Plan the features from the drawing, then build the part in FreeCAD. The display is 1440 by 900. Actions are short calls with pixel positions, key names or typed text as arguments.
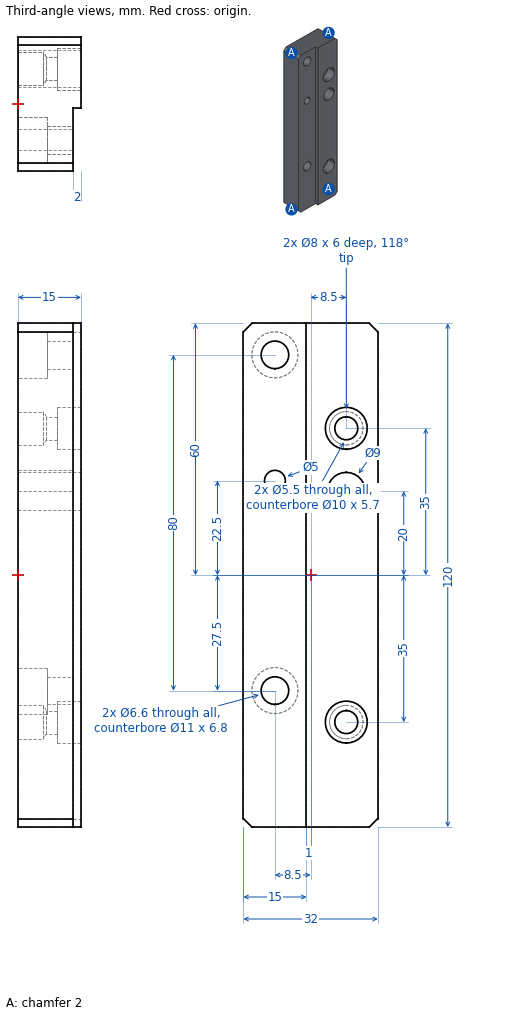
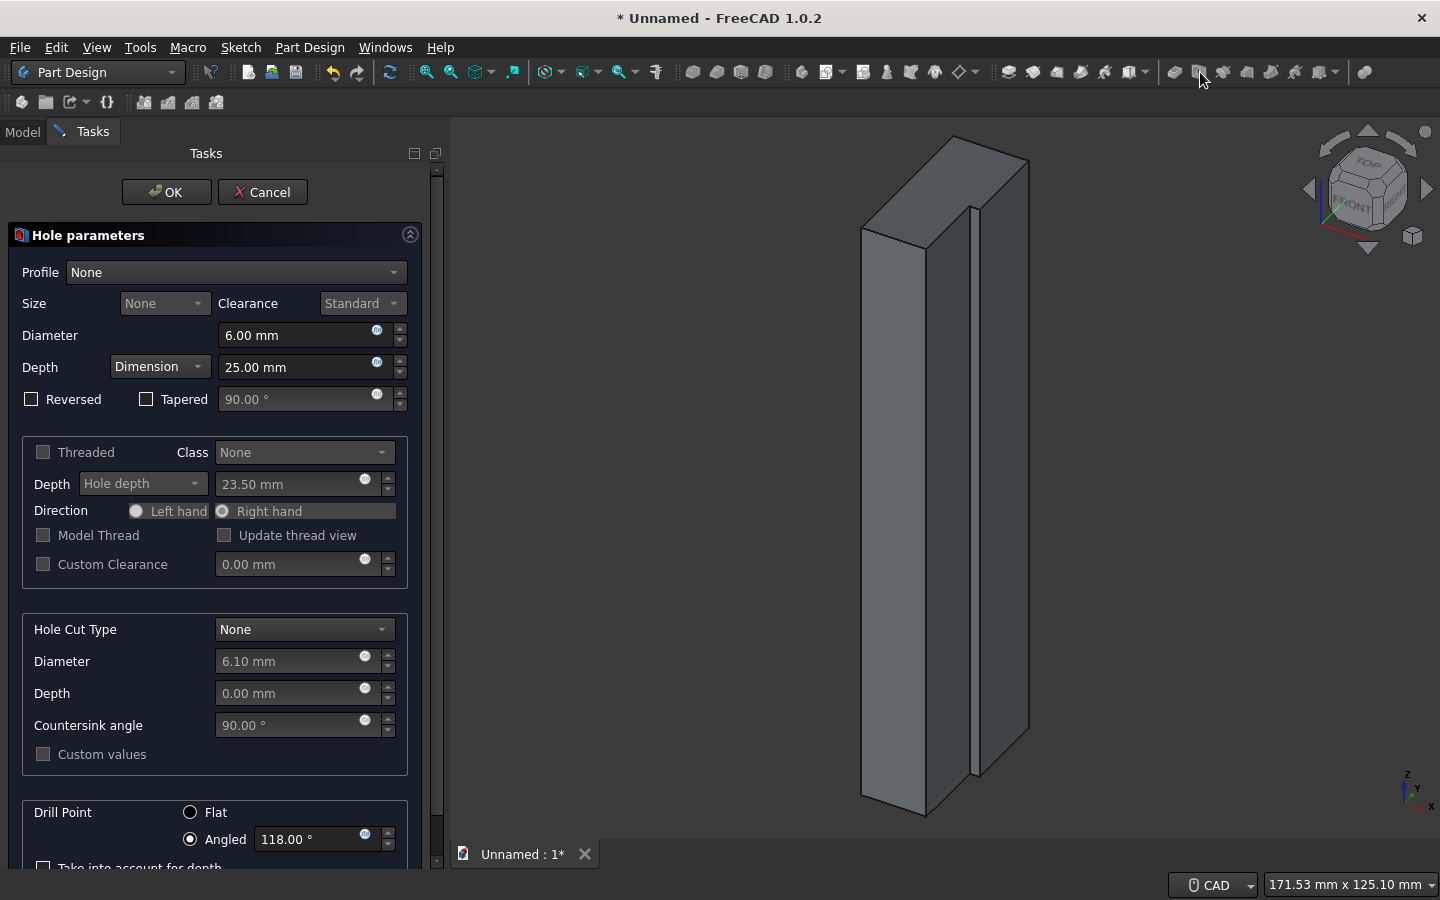
triple_click(305, 335)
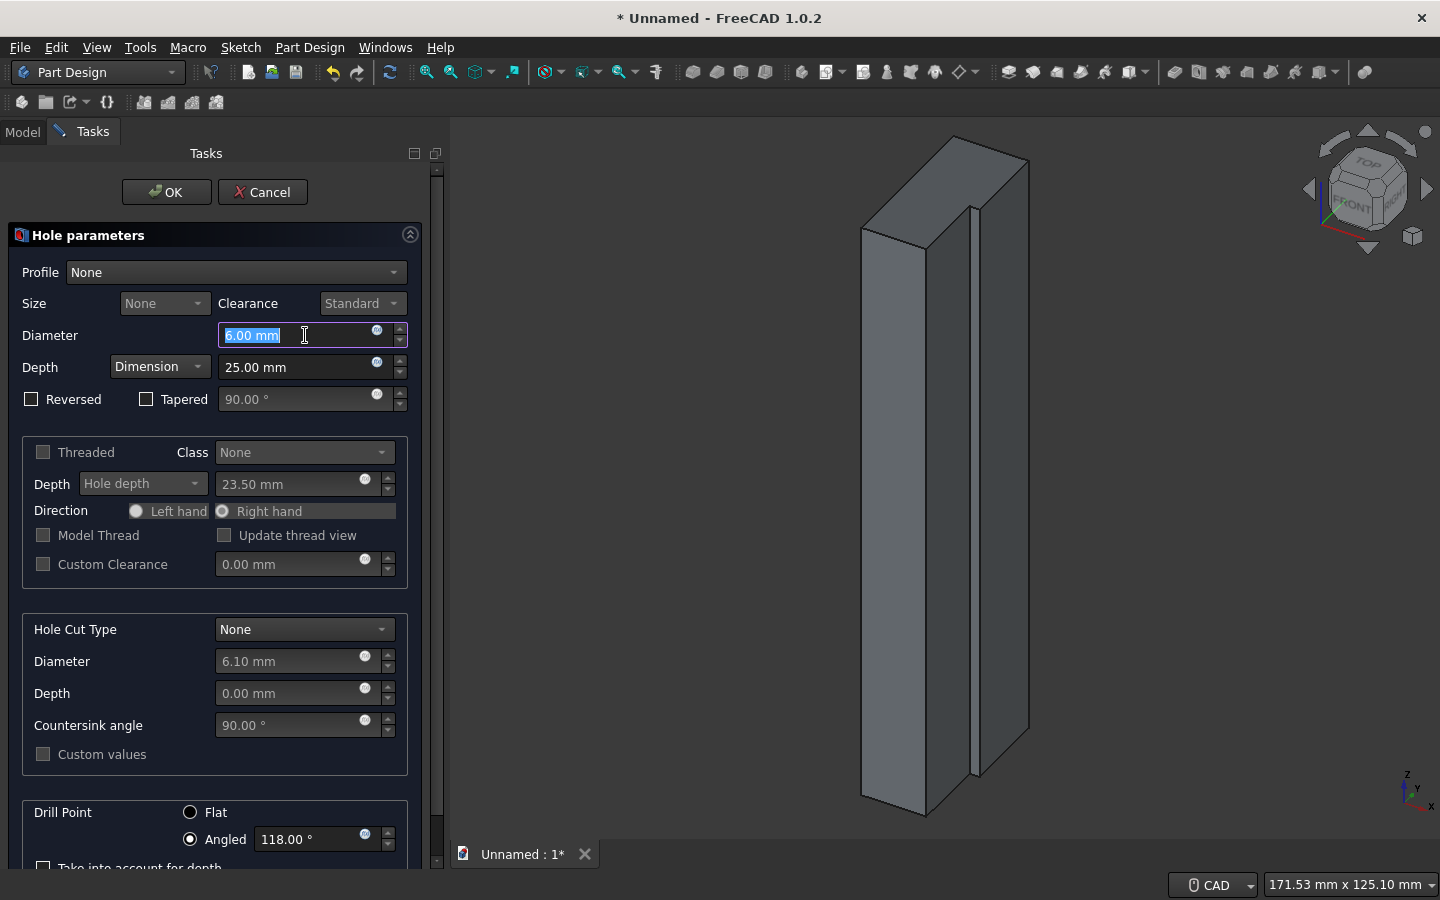
text(8)
key(Tab)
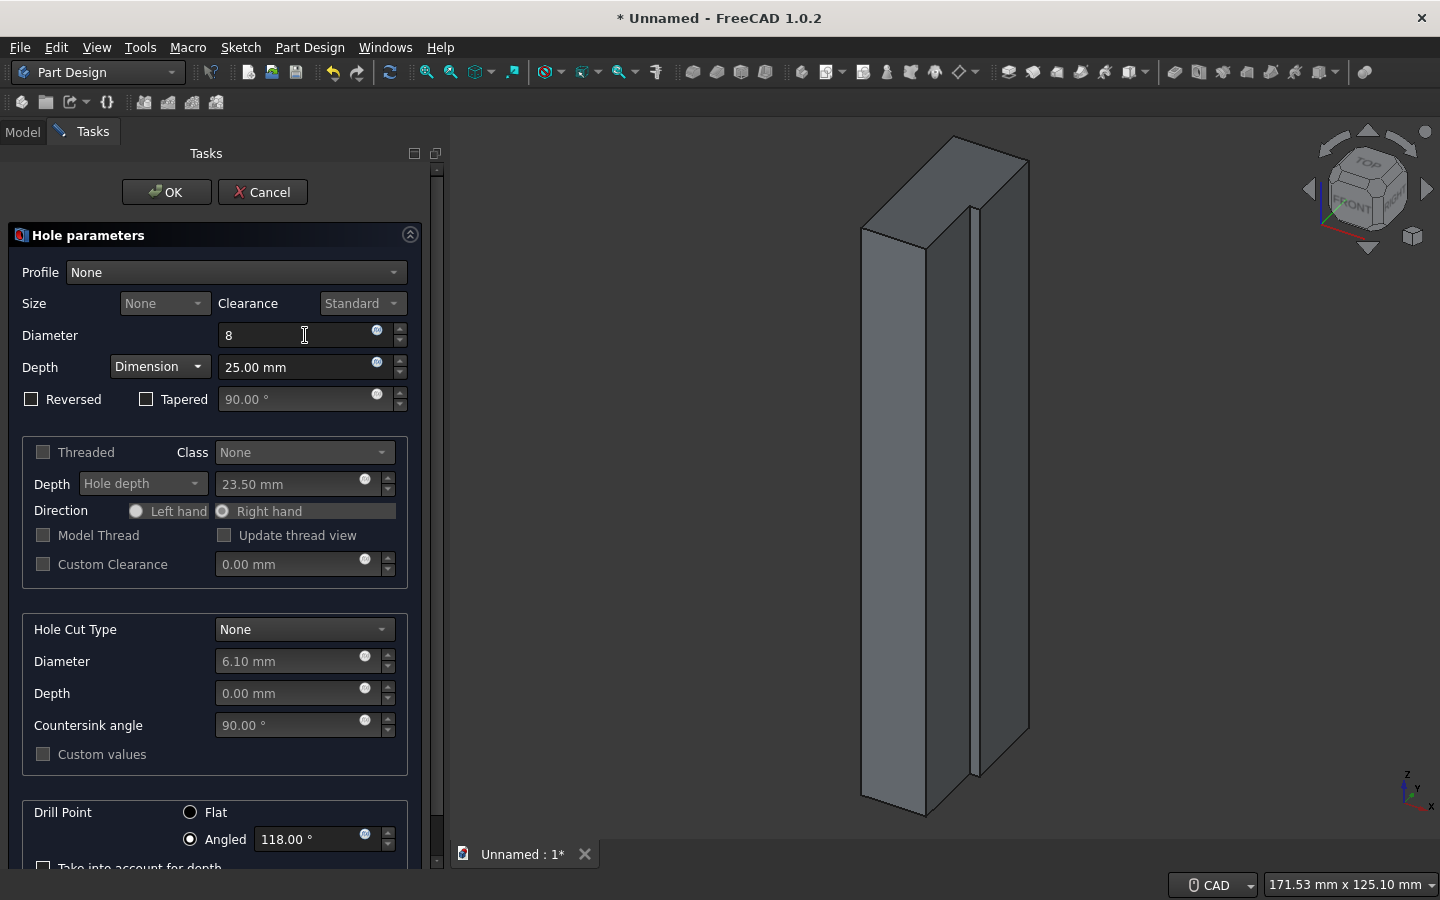
triple_click(305, 367)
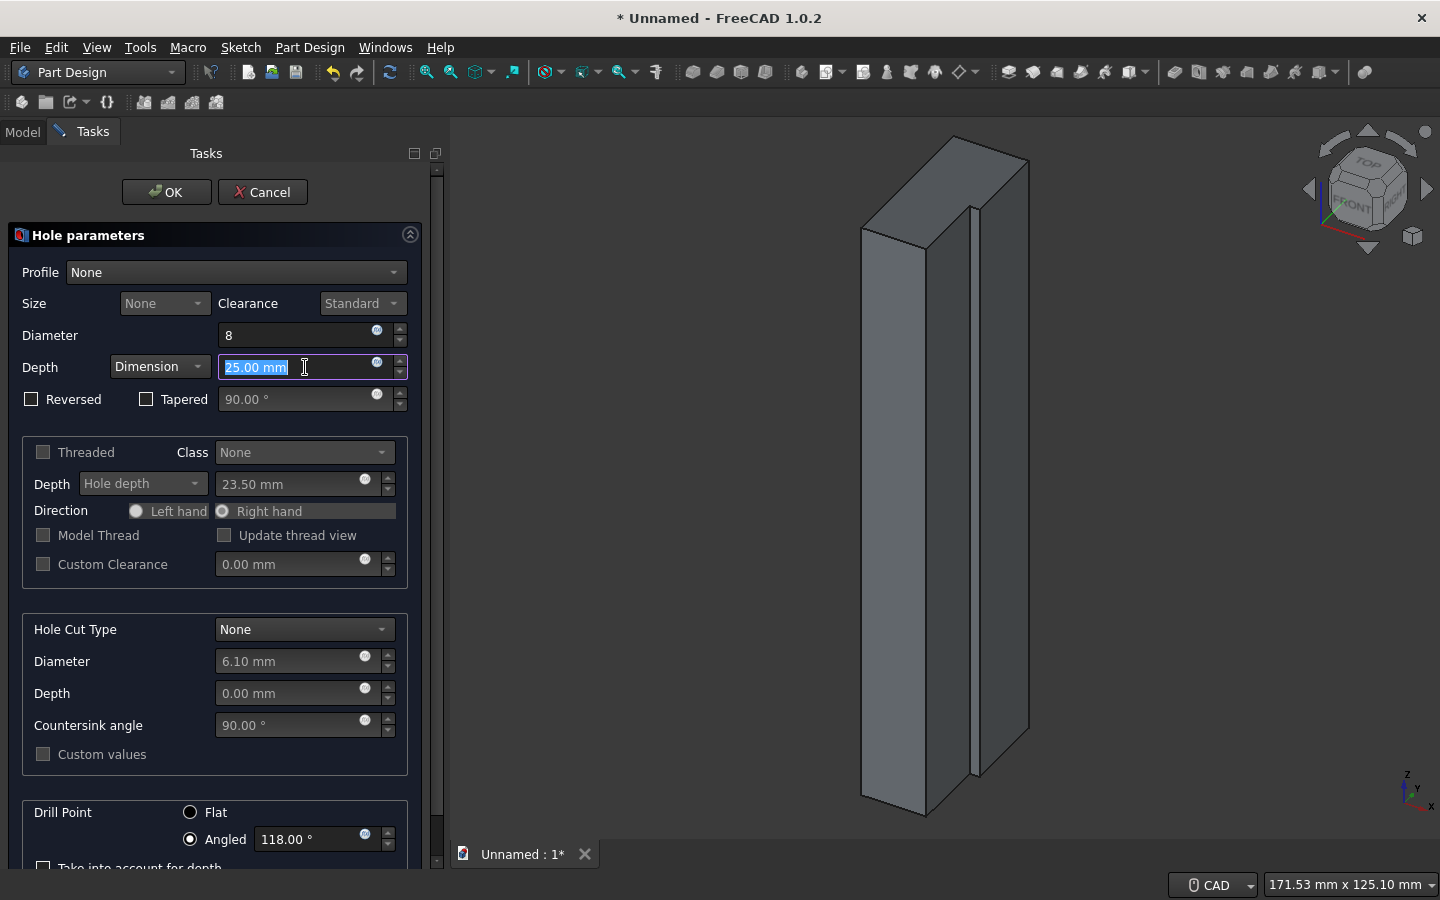
text(6)
key(Tab)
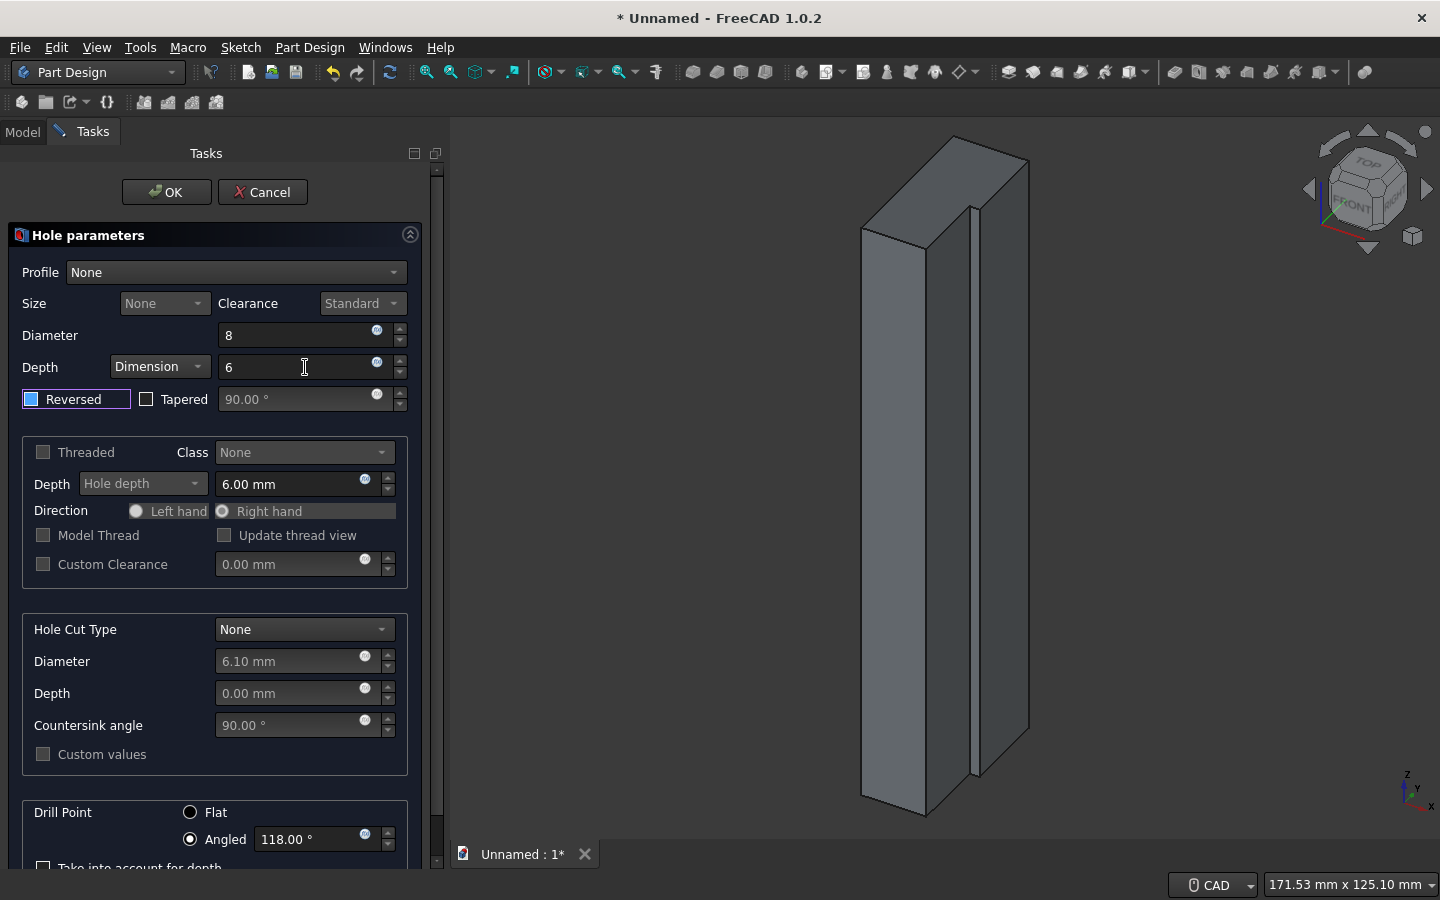
click(30, 399)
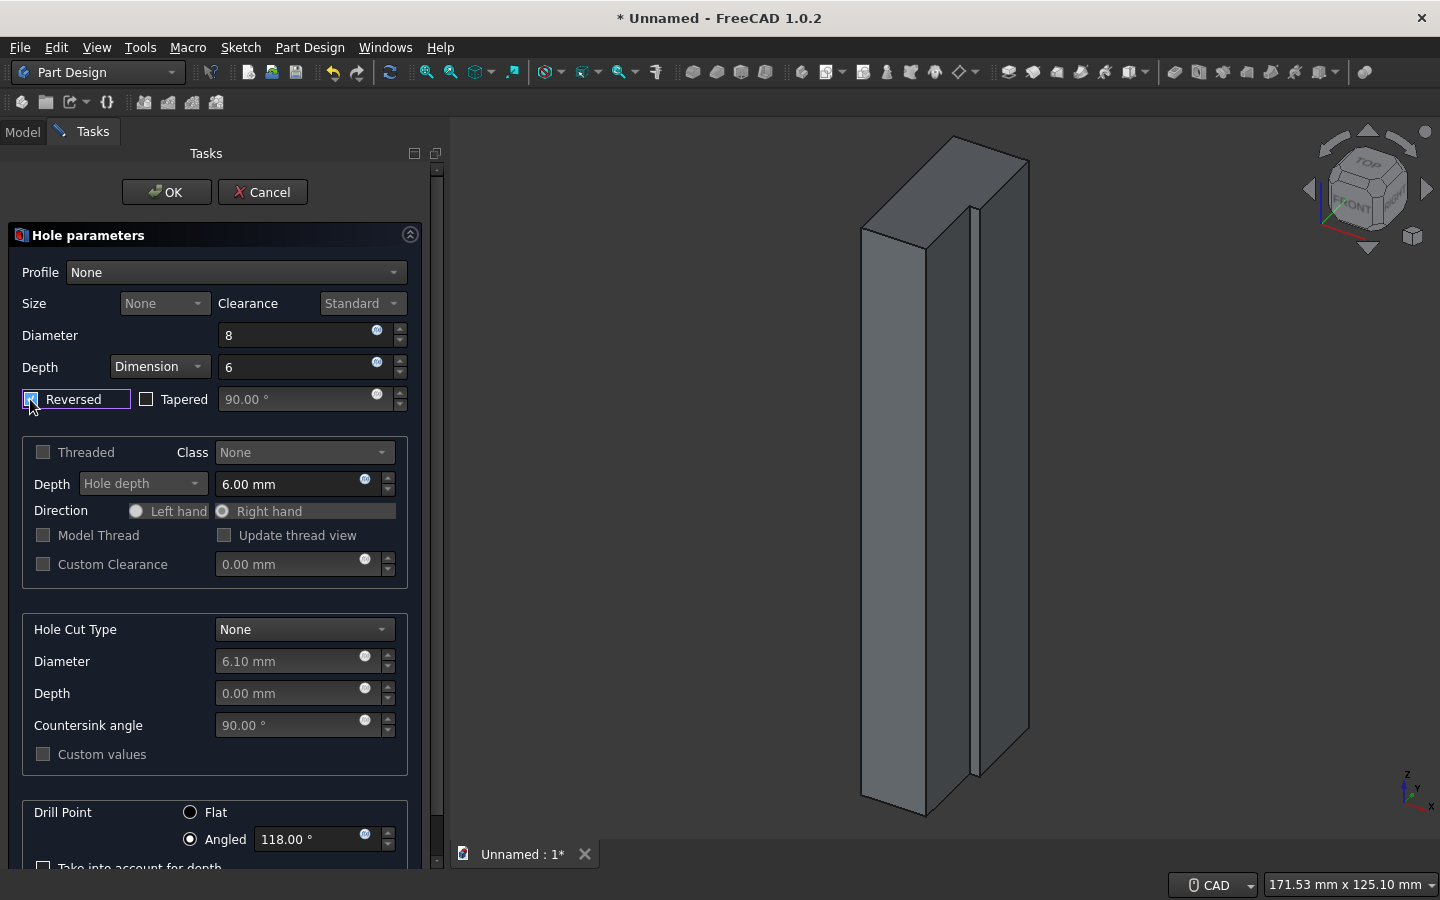
click(167, 192)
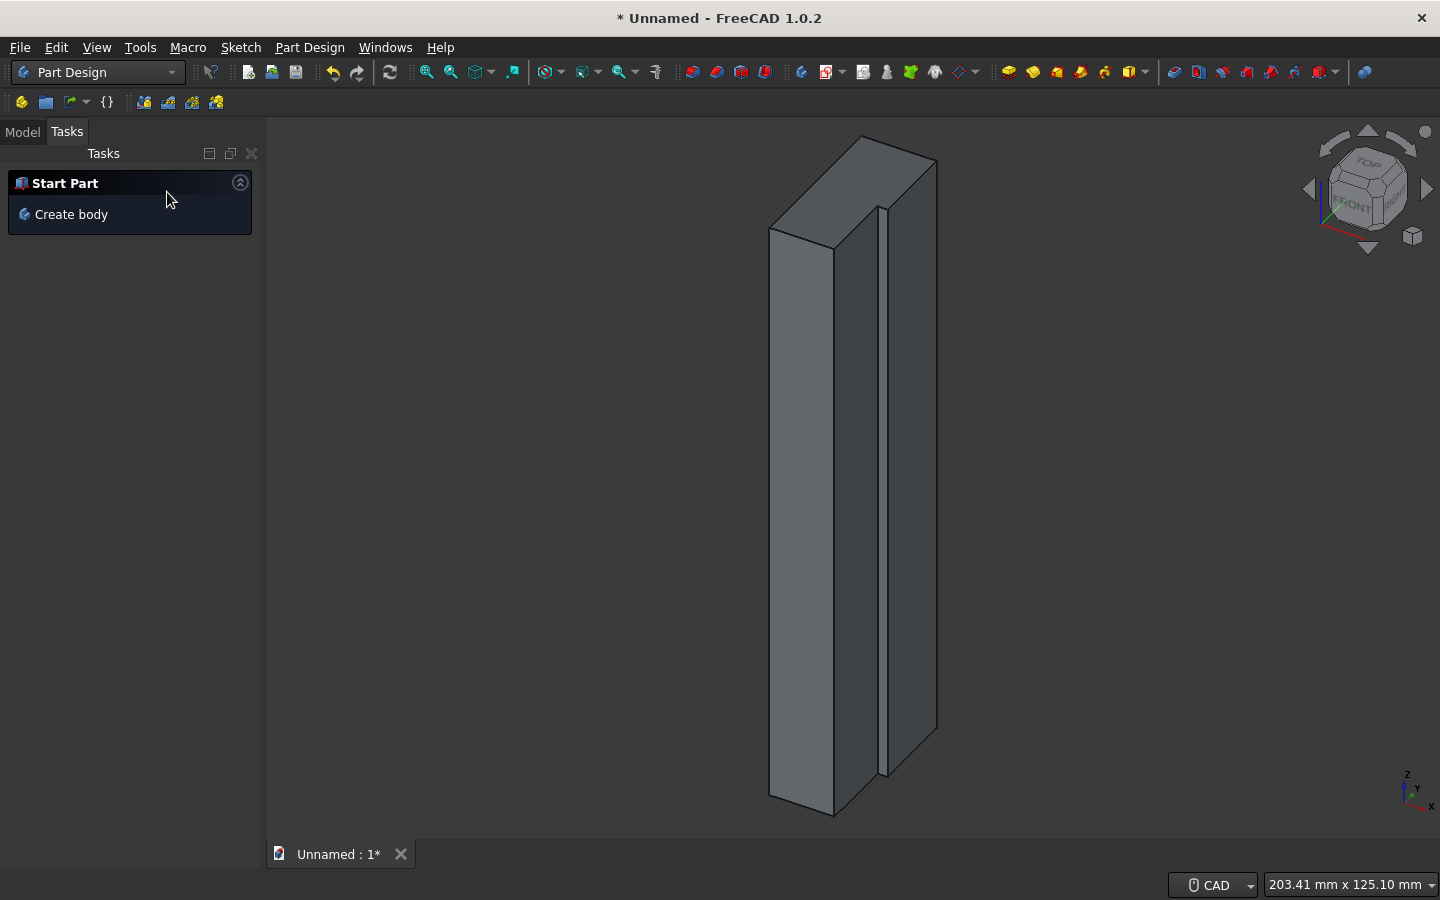
click(912, 306)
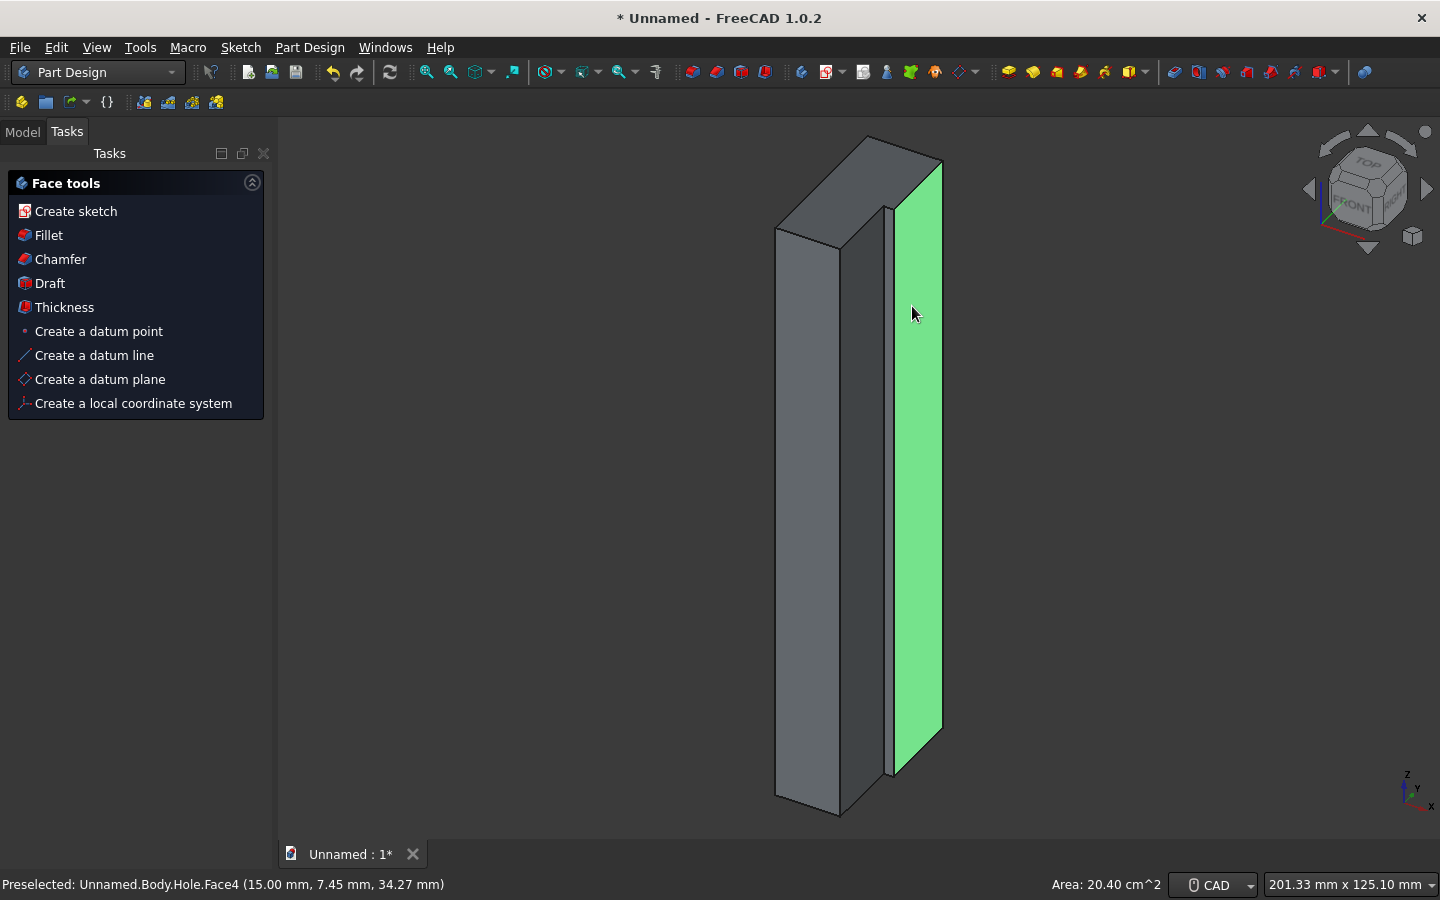
click(826, 72)